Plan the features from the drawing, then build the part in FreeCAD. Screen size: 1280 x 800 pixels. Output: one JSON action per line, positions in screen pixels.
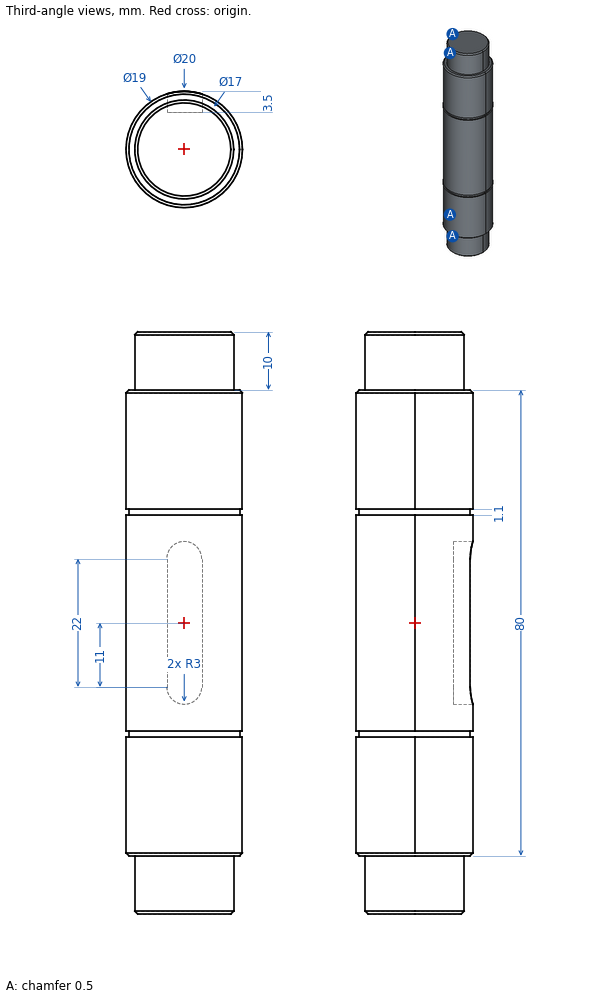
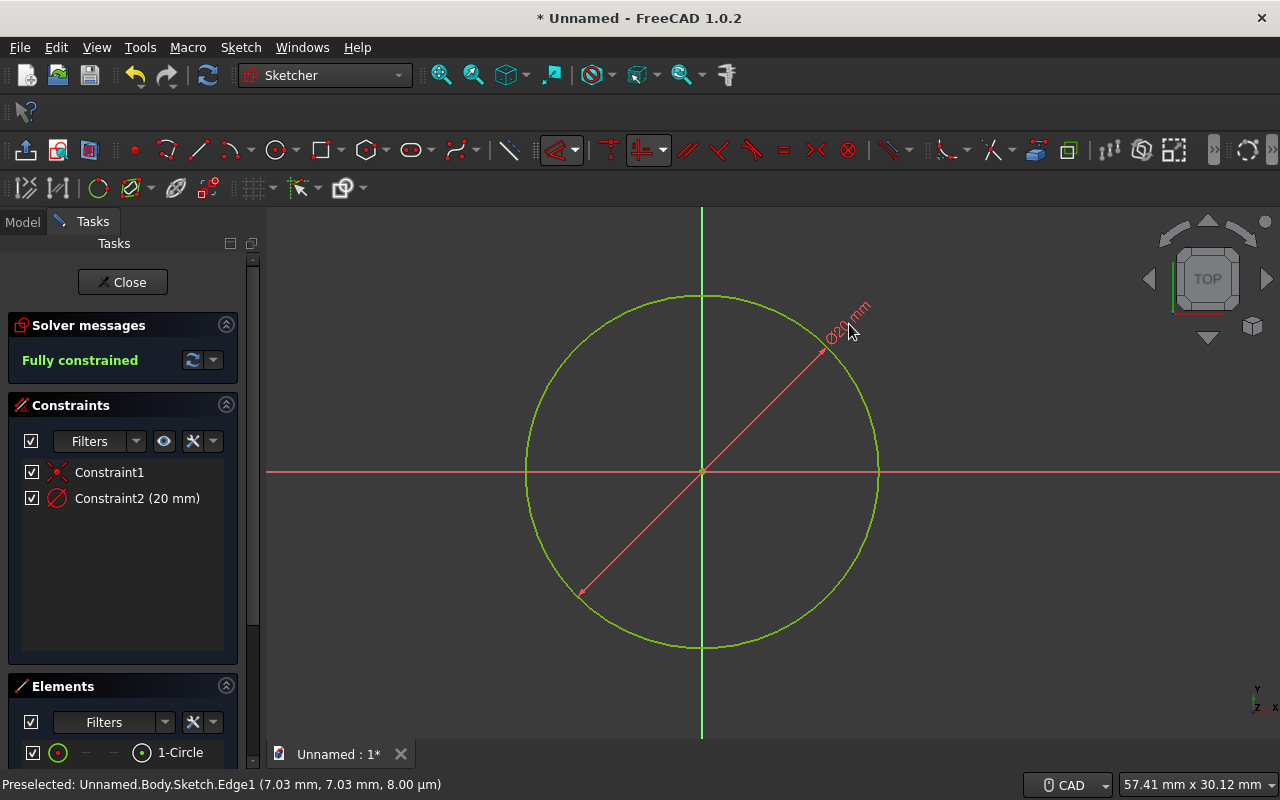
{"action": "left_click", "coordinate": [123, 282]}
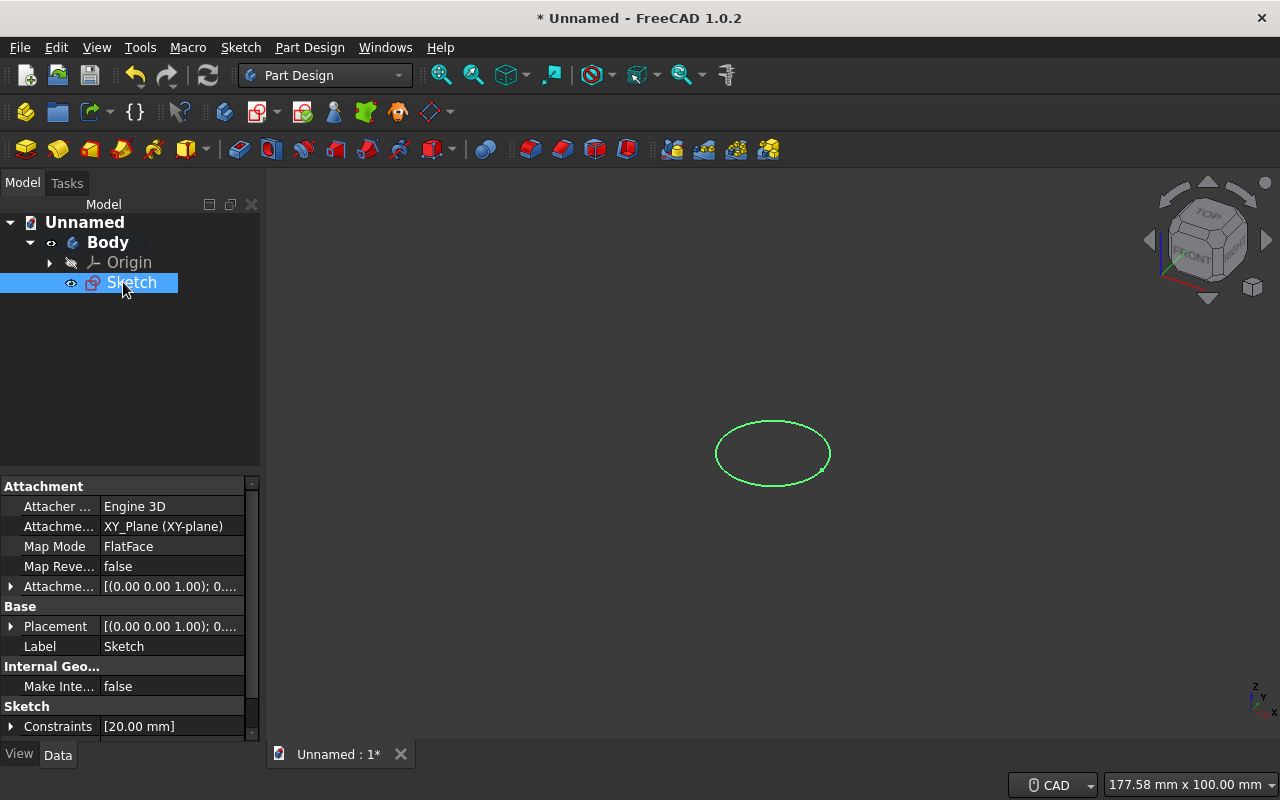
{"action": "left_click", "coordinate": [26, 150]}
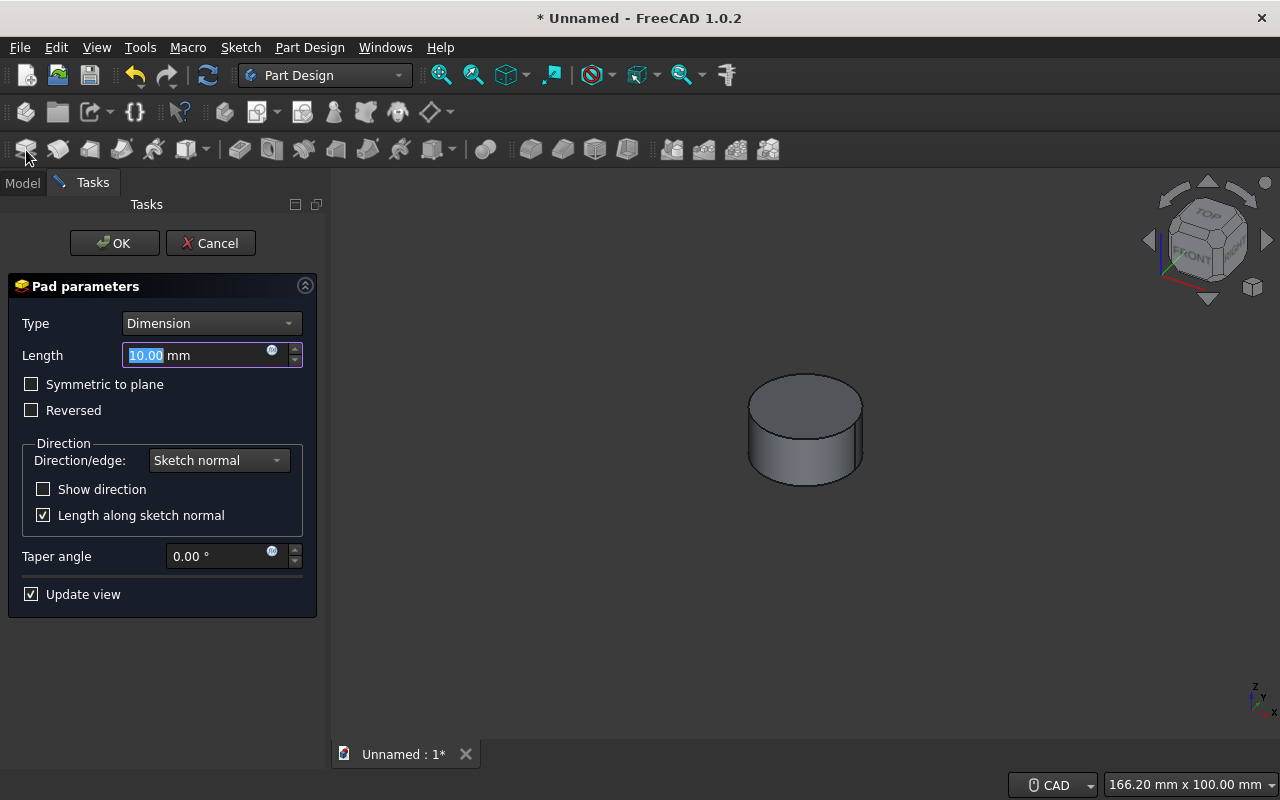
{"action": "type", "text": "80"}
{"action": "key", "text": "Tab"}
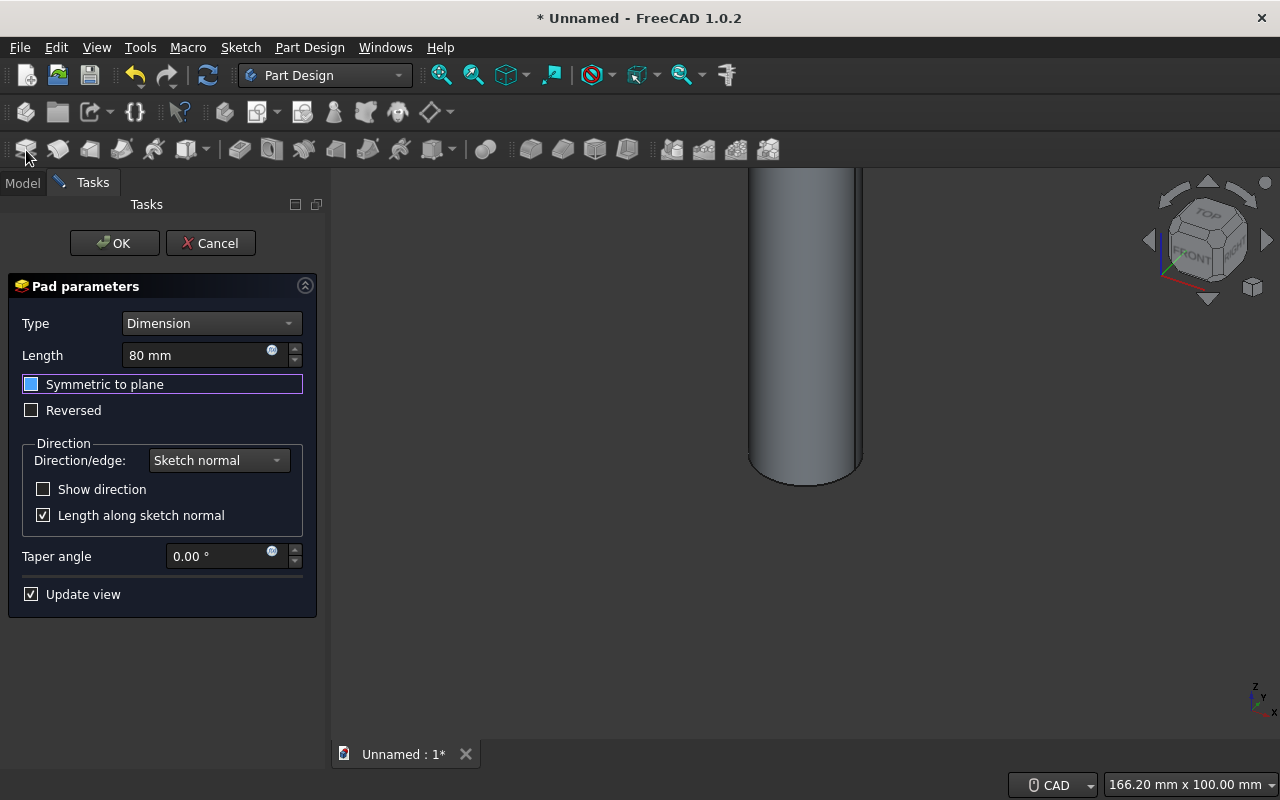
{"action": "left_click", "coordinate": [30, 384]}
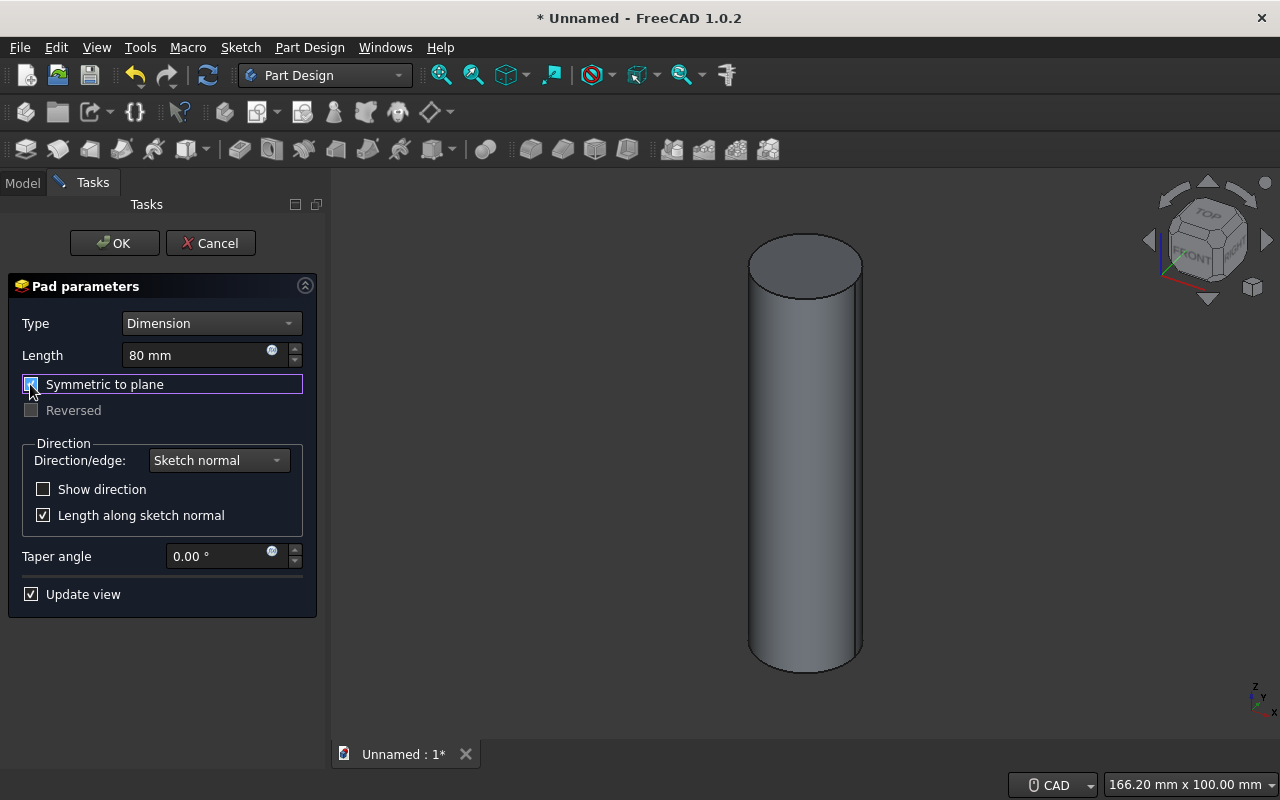
{"action": "left_click", "coordinate": [115, 243]}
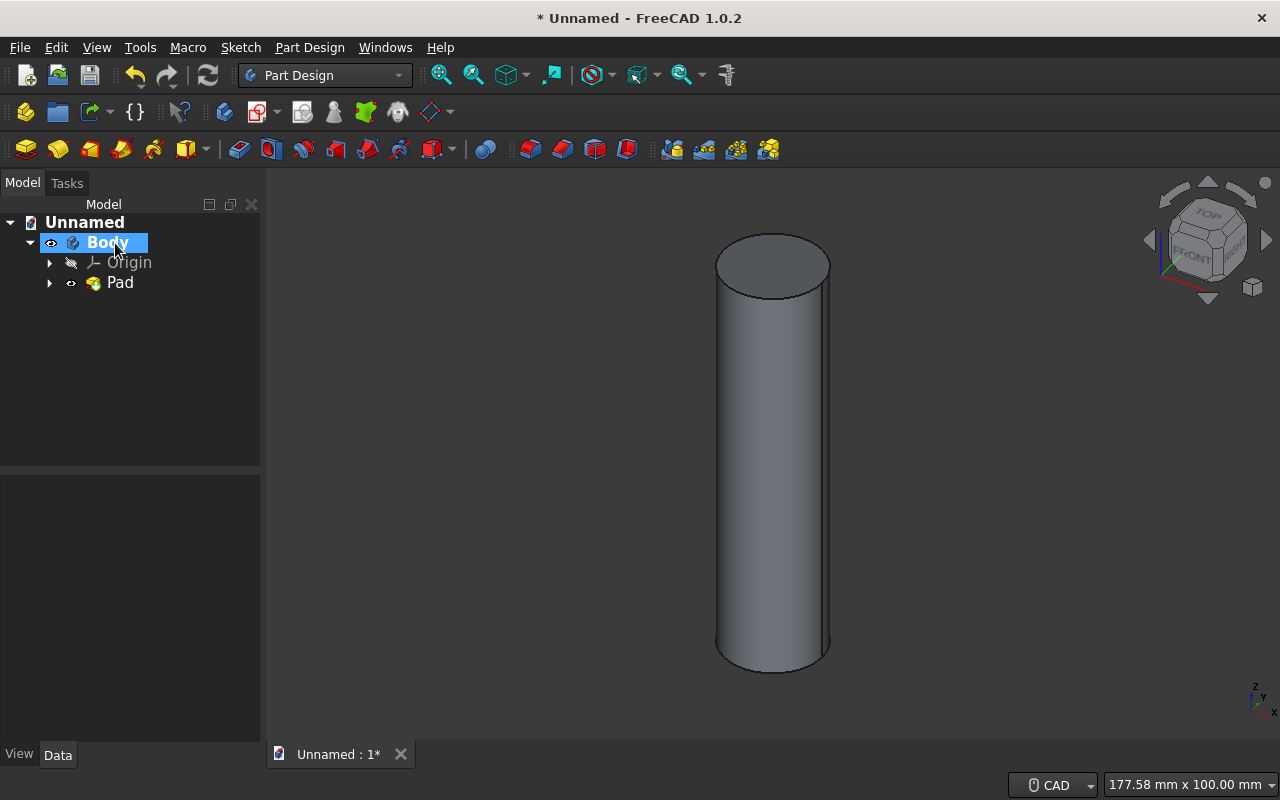
{"action": "left_click", "coordinate": [773, 265]}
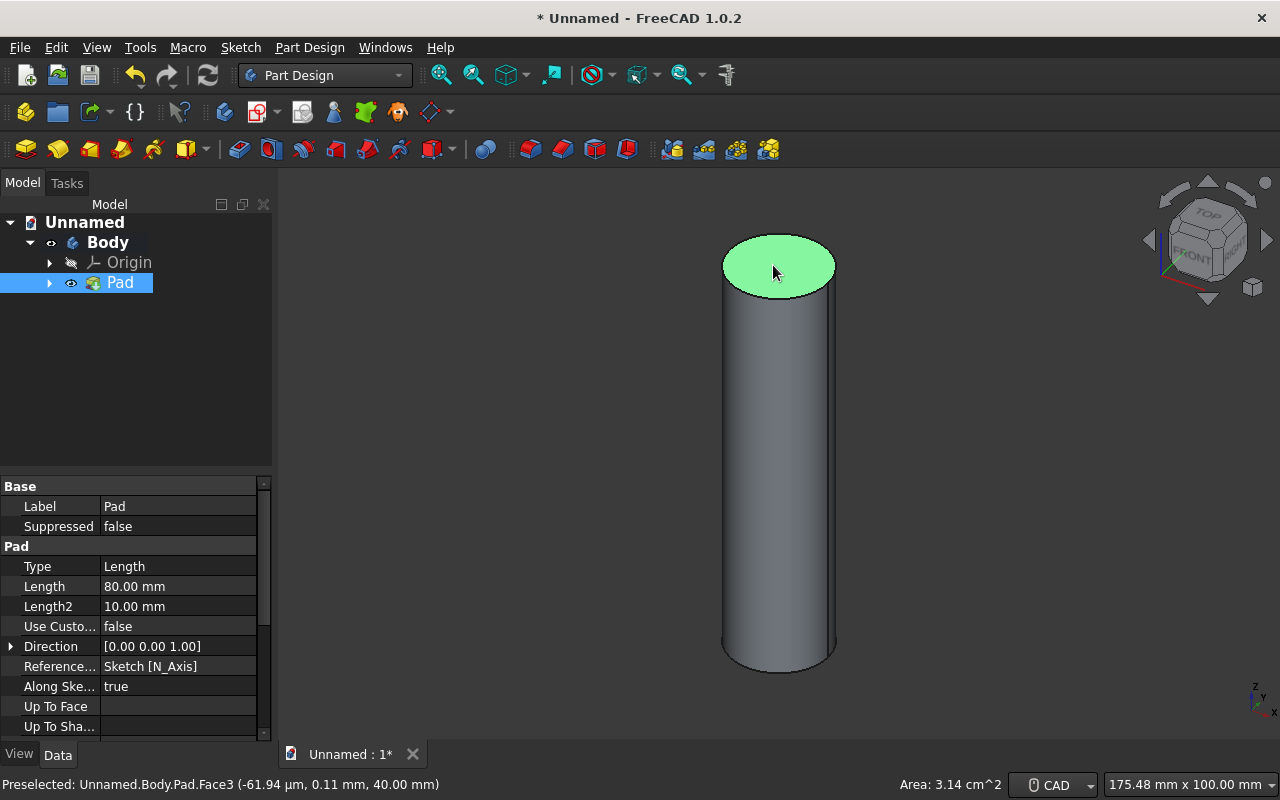
{"action": "left_click", "coordinate": [258, 112]}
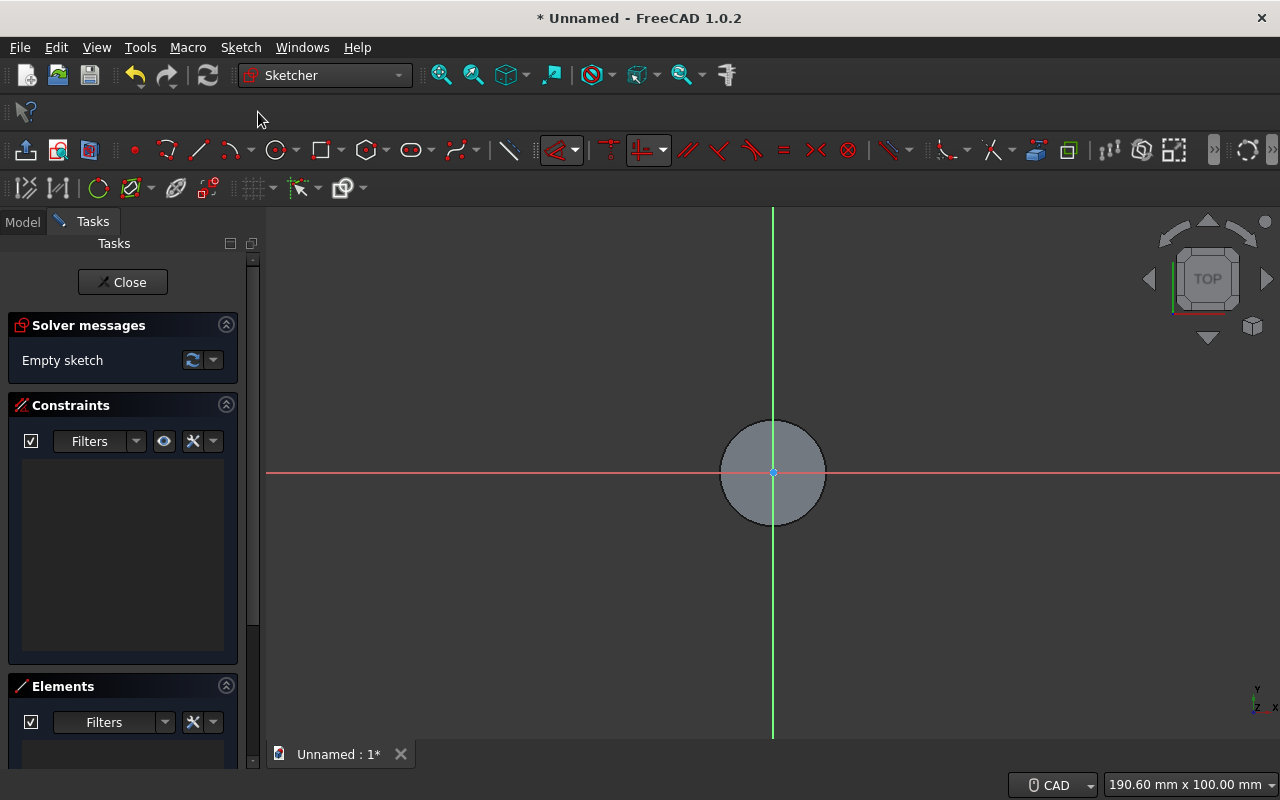
{"action": "scroll", "coordinate": [795, 473], "scroll_direction": "up", "scroll_amount": 7}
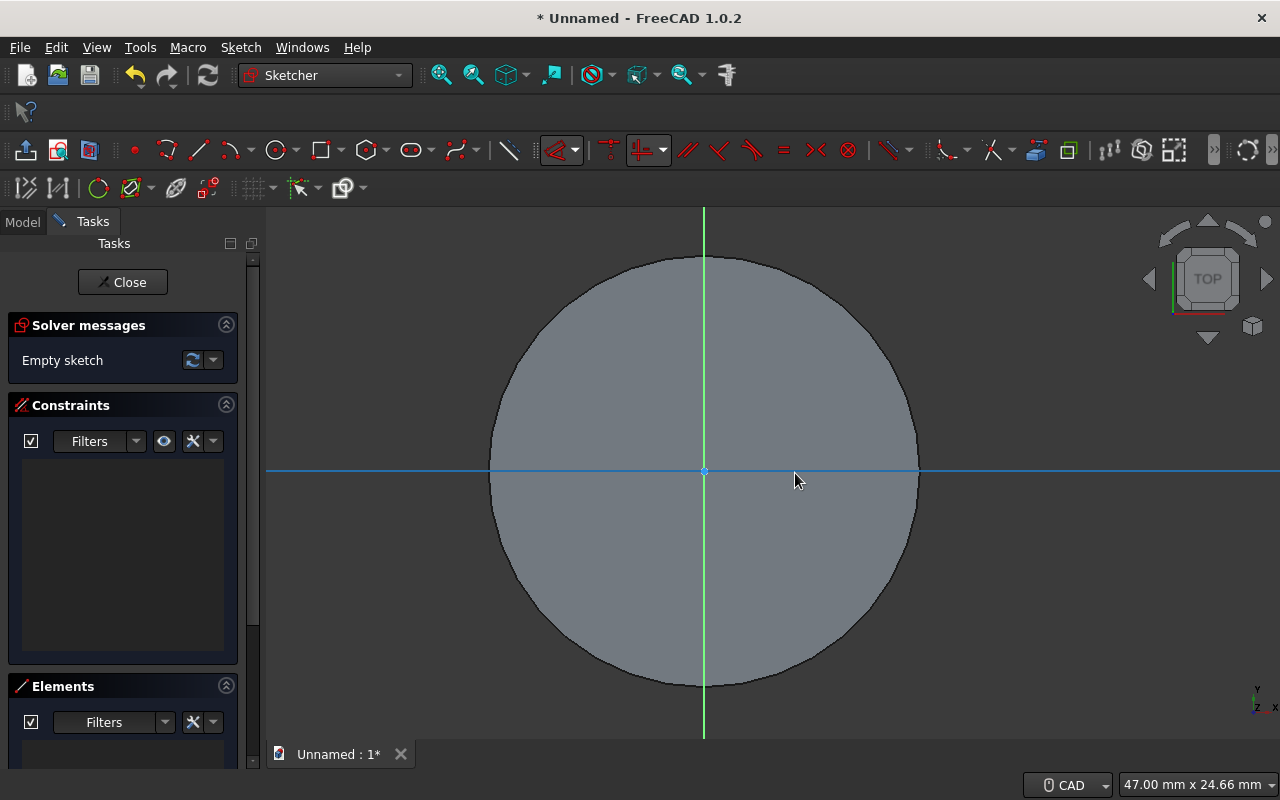
{"action": "key", "text": "g c"}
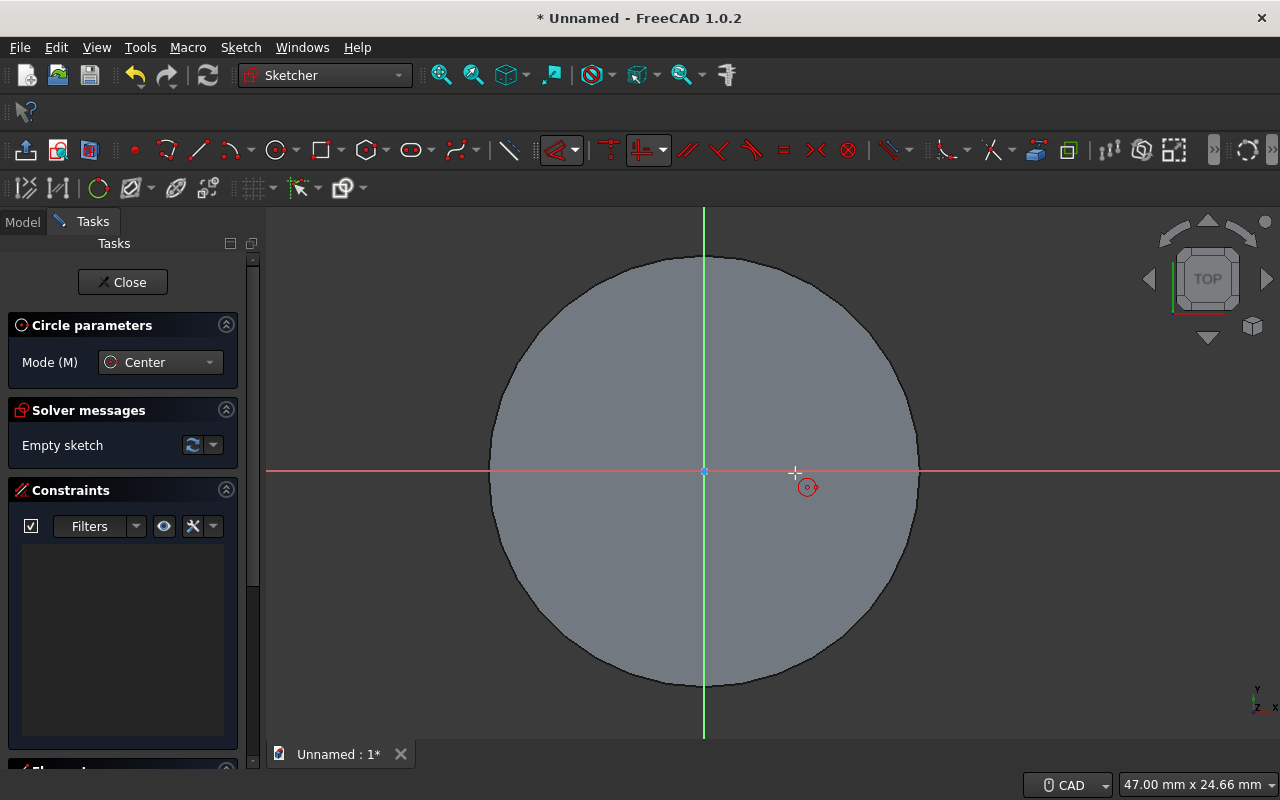
{"action": "left_click", "coordinate": [704, 471]}
{"action": "left_click", "coordinate": [834, 342]}
{"action": "key", "text": "Escape"}